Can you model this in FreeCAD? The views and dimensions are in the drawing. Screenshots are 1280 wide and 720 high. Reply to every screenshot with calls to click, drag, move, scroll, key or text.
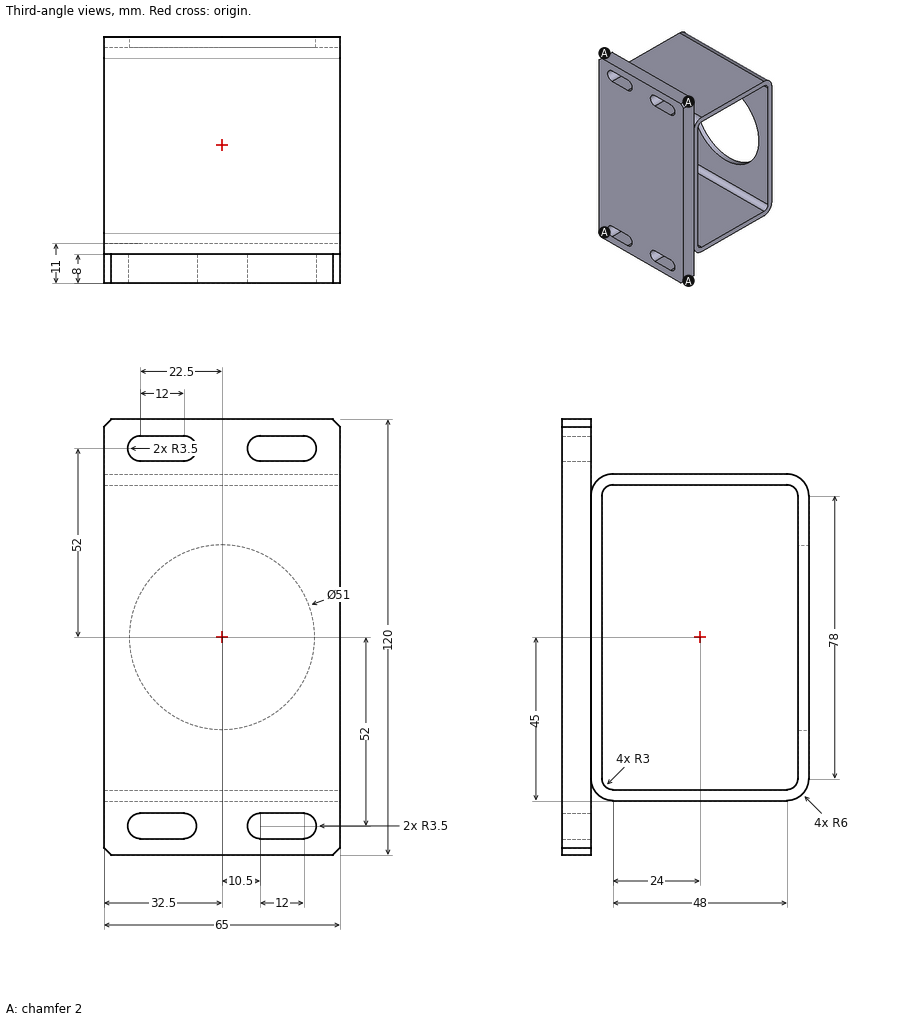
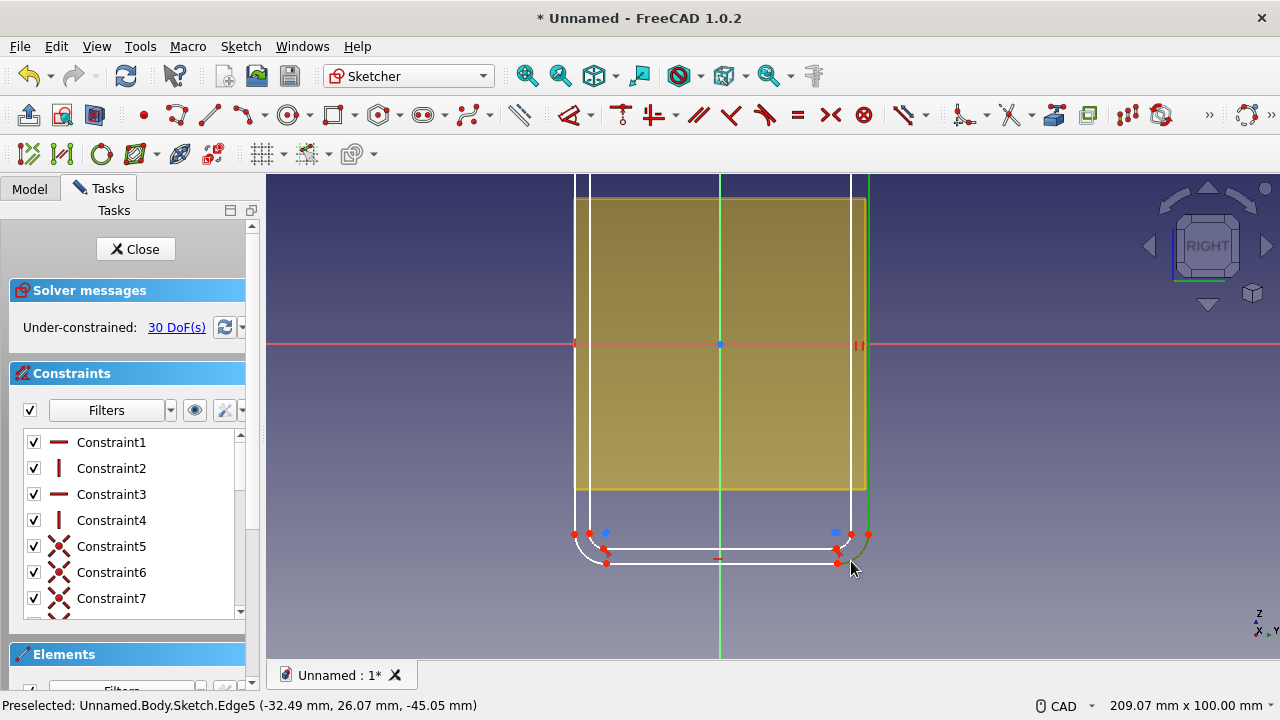
click(765, 116)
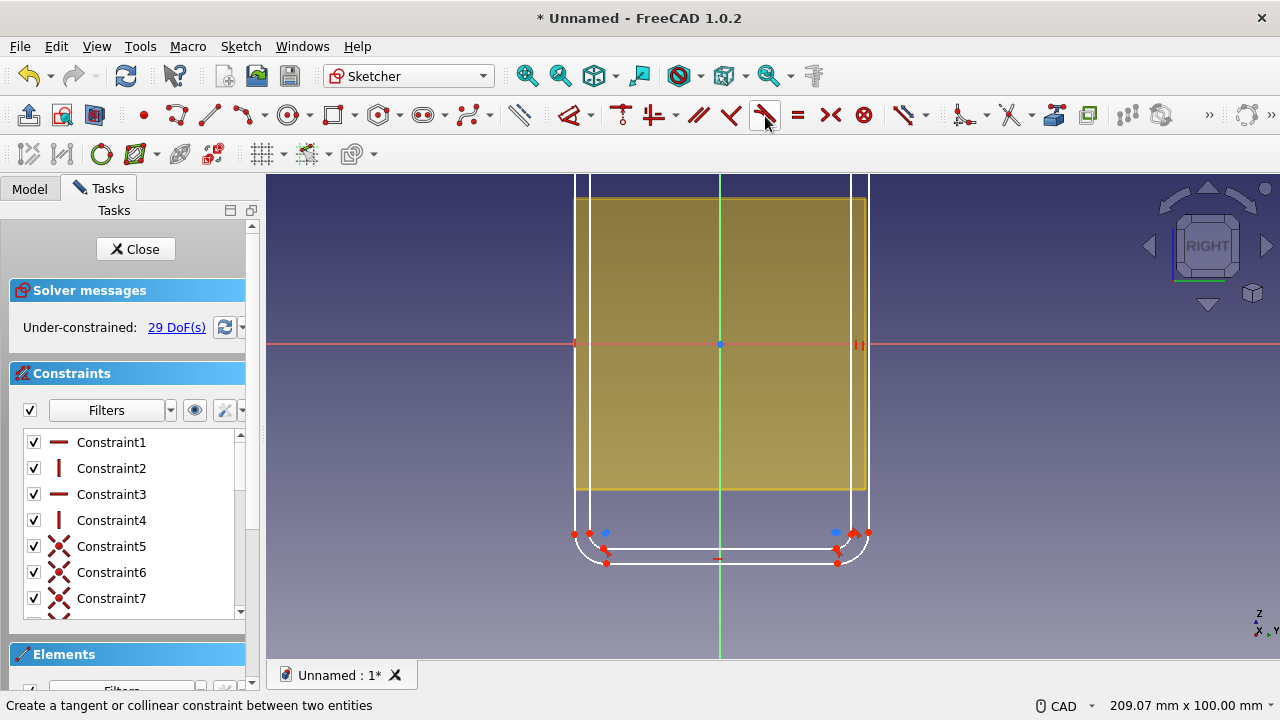
click(869, 420)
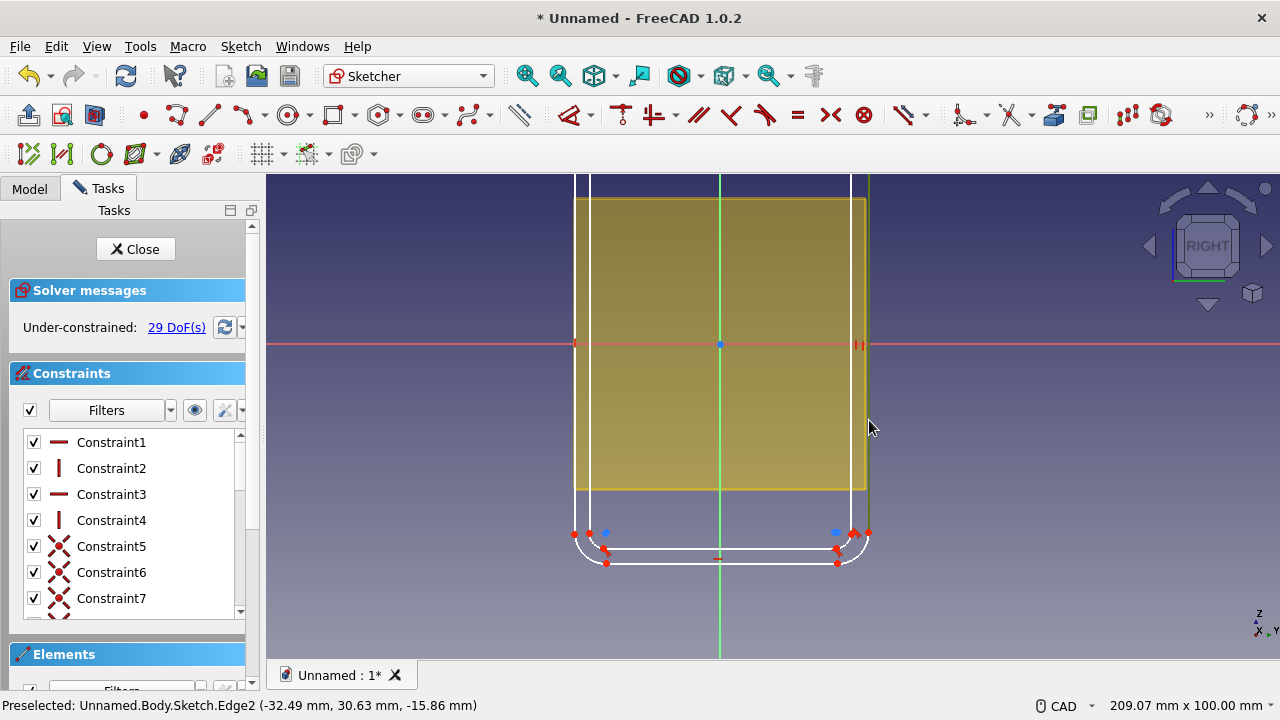
scroll(673, 564, down, 2)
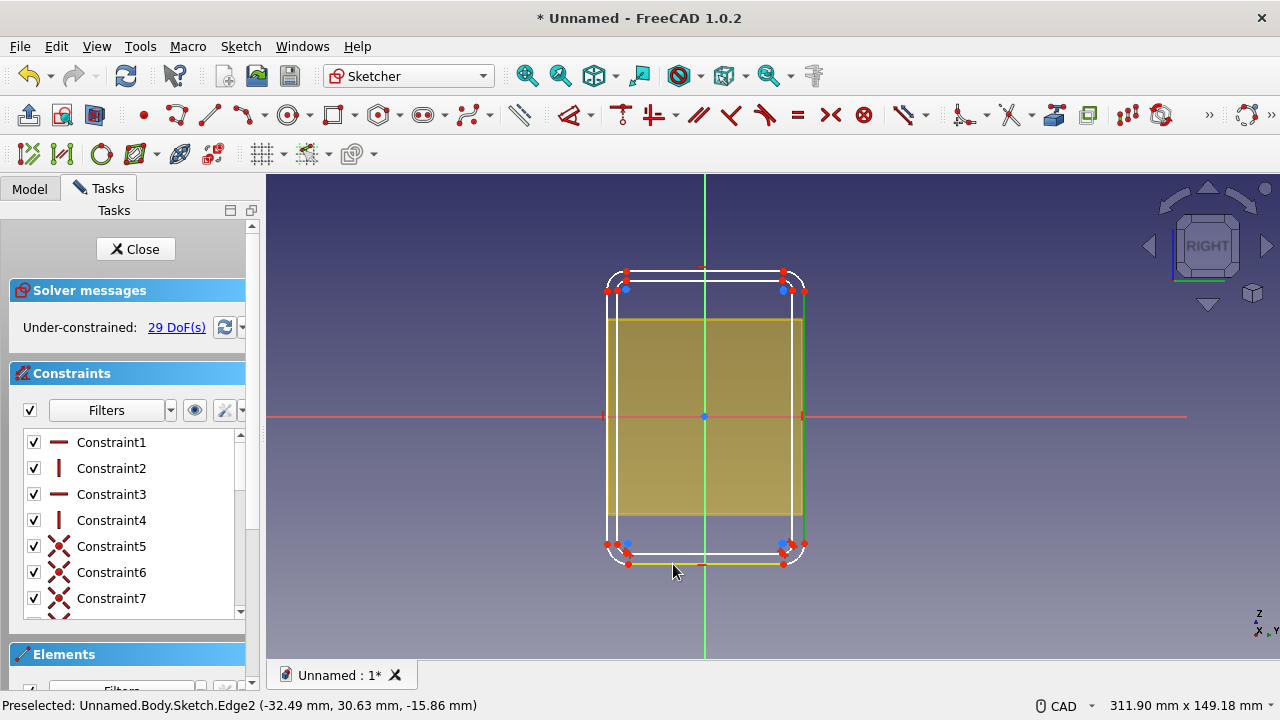
scroll(802, 282, up, 2)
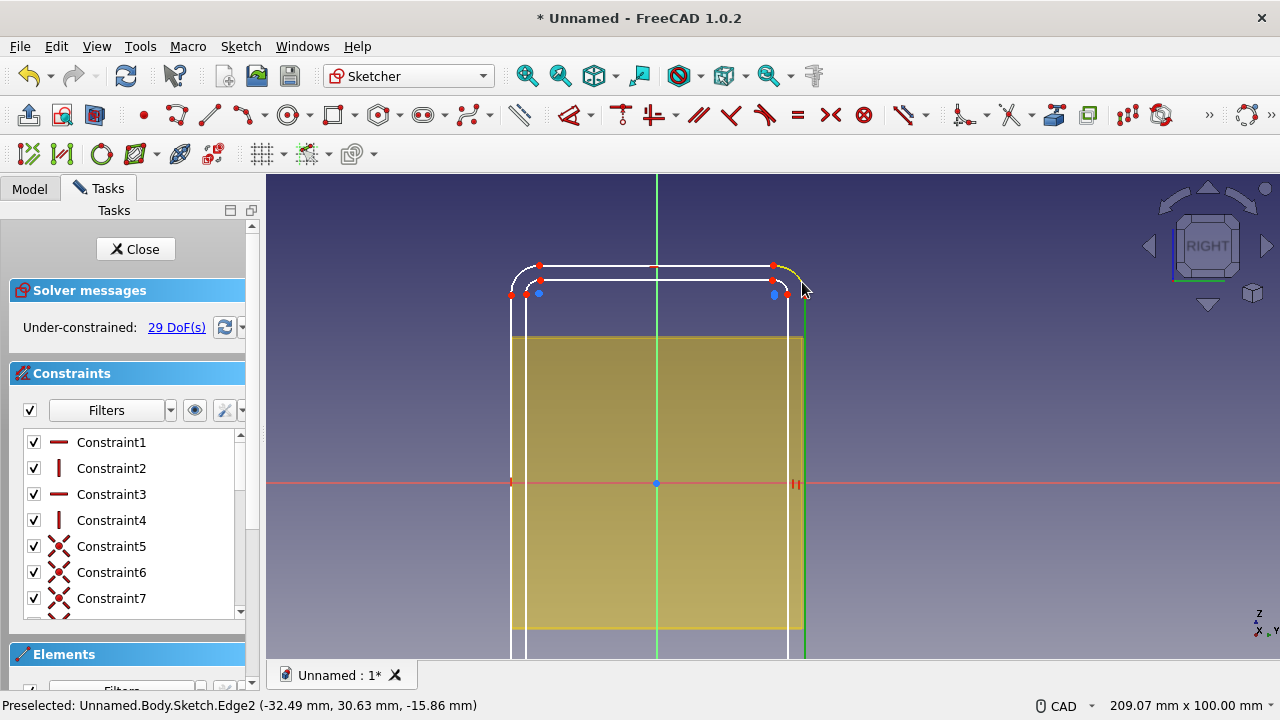
click(802, 282)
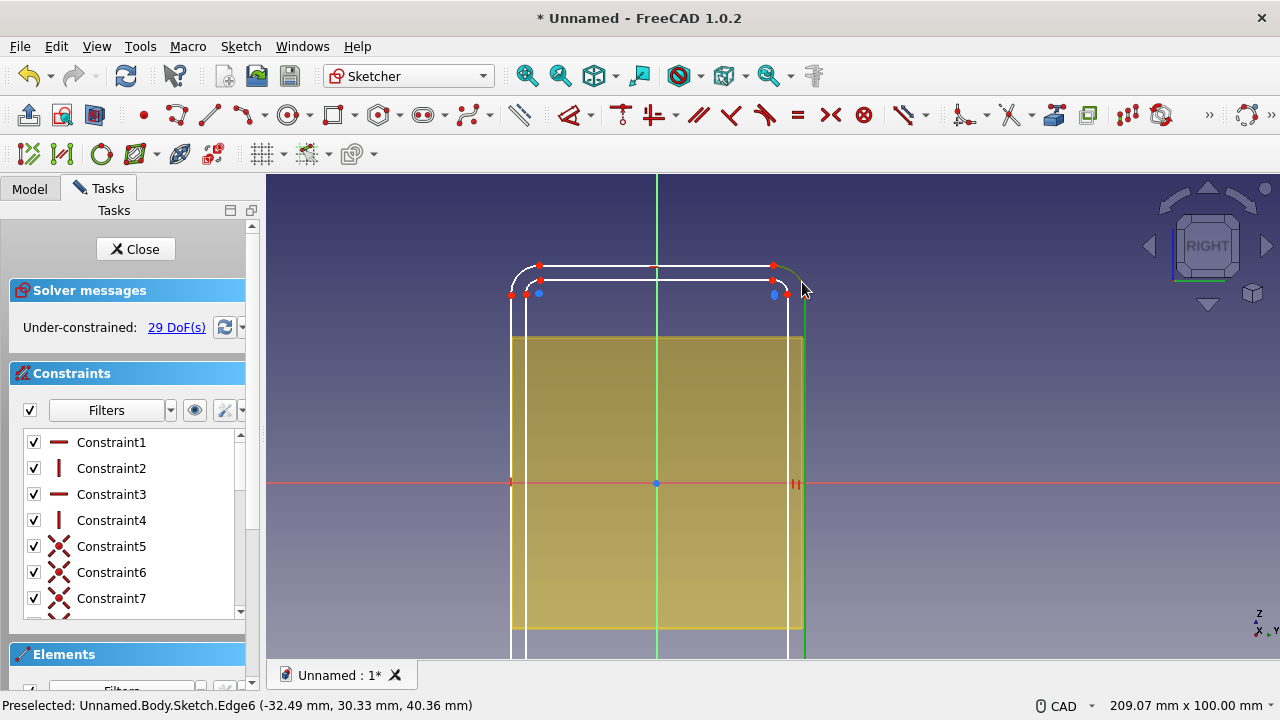
click(765, 116)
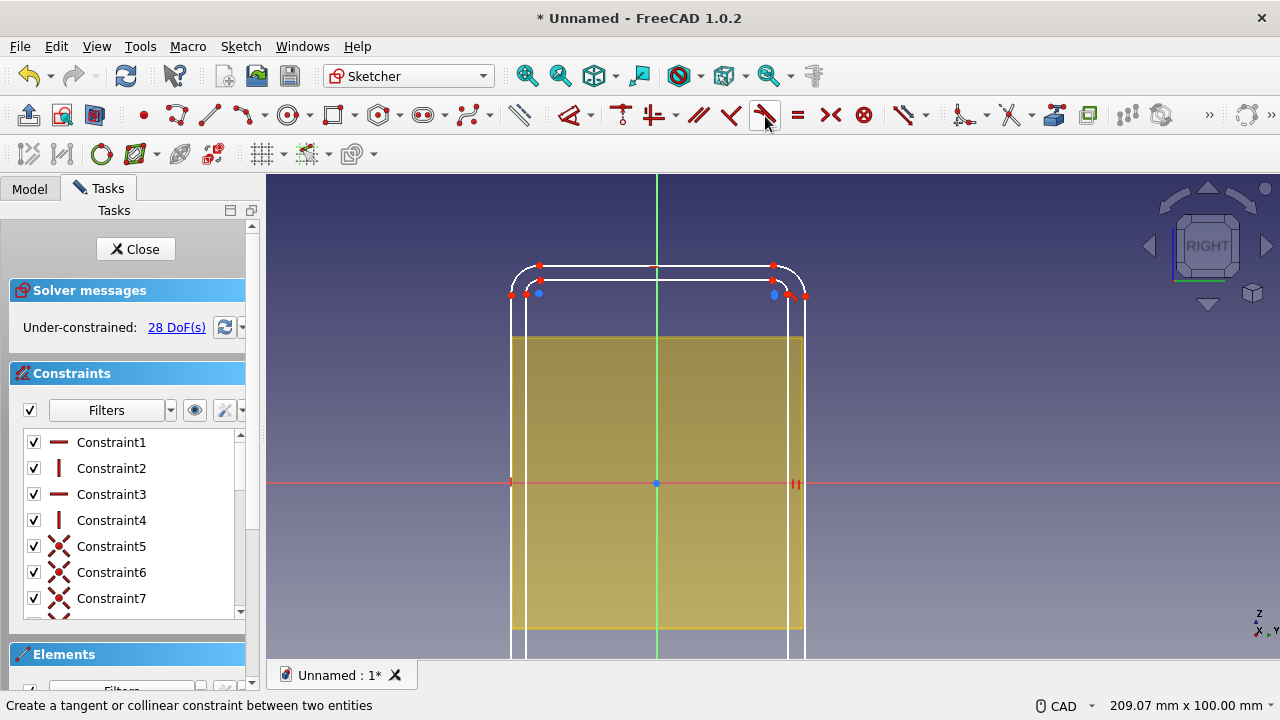
click(703, 266)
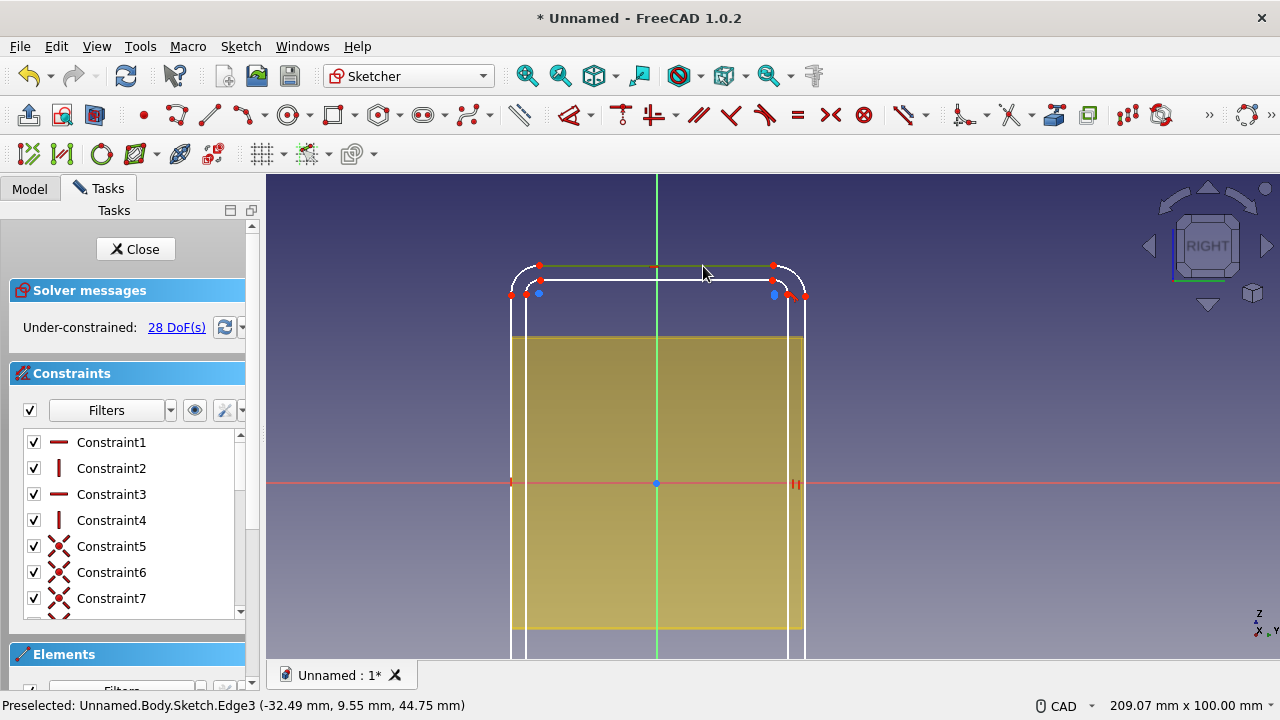
click(802, 282)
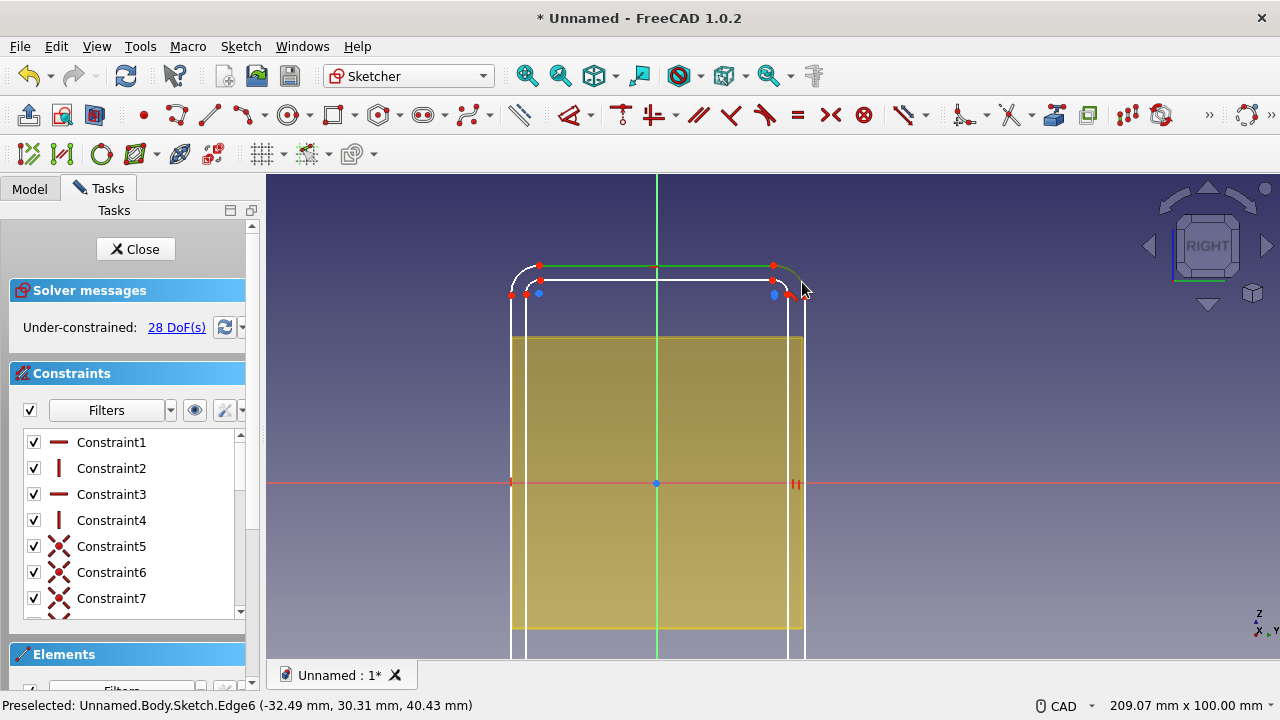
click(765, 116)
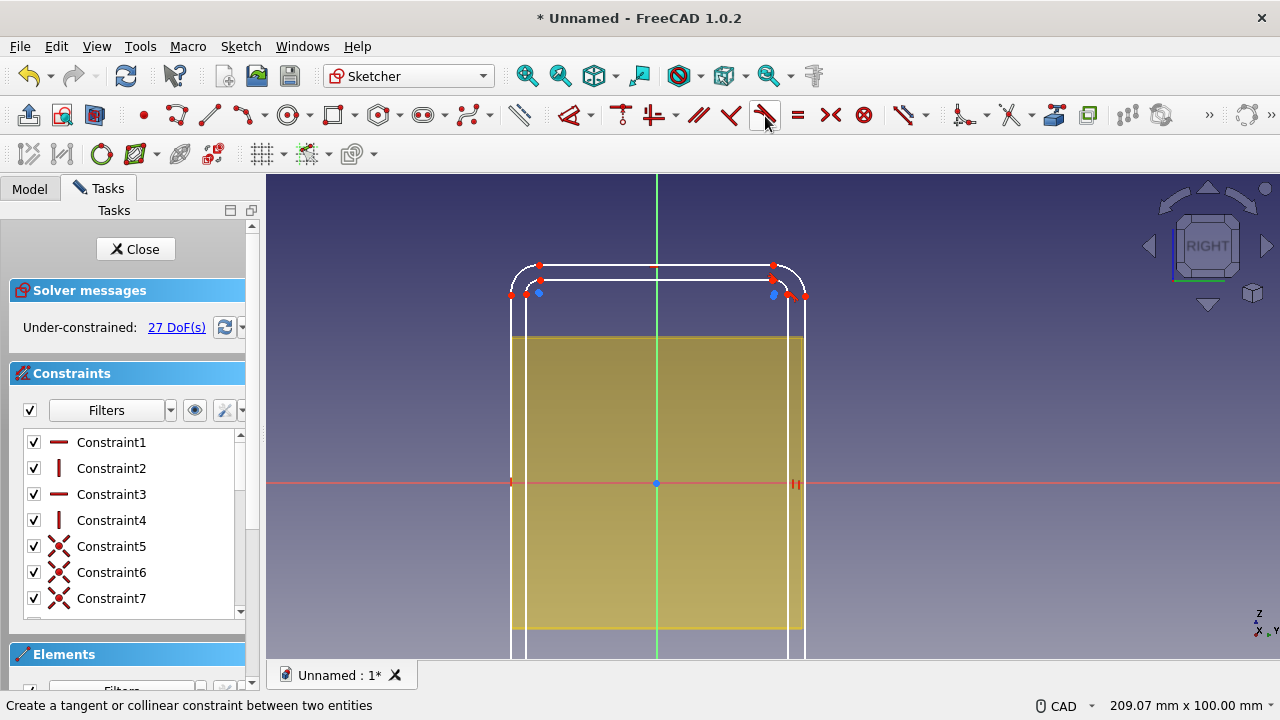
click(703, 265)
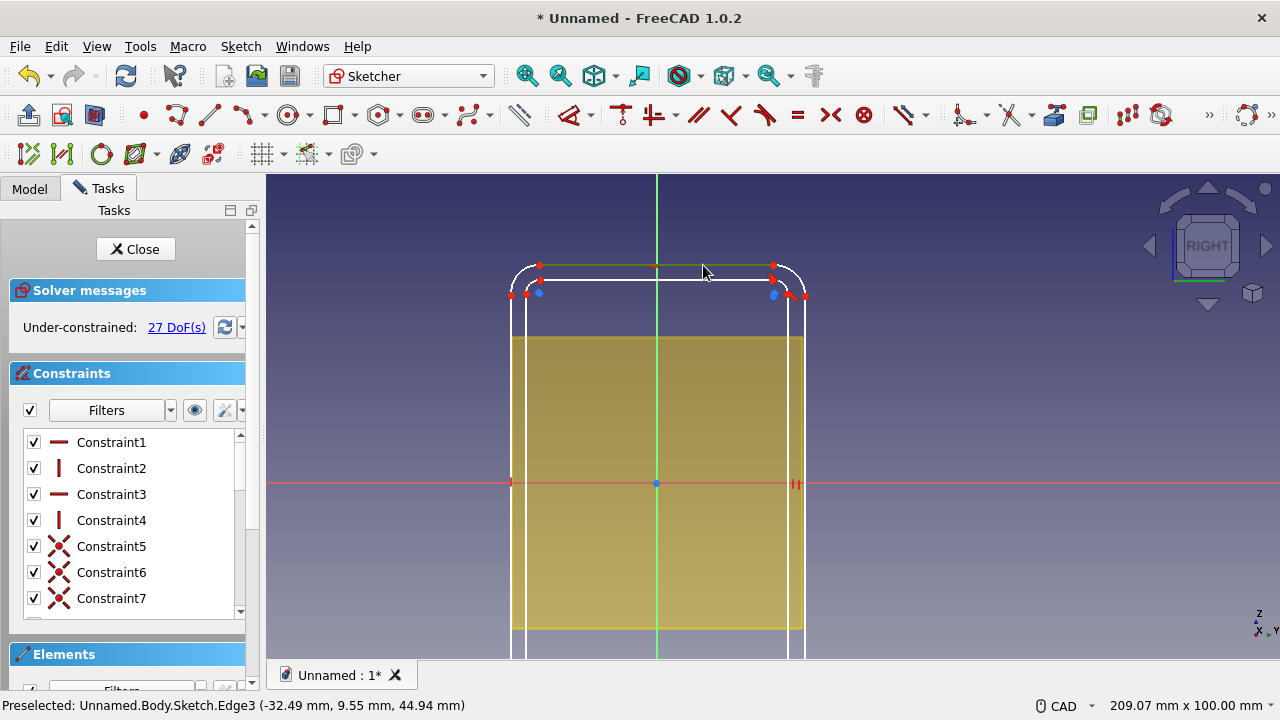
click(526, 268)